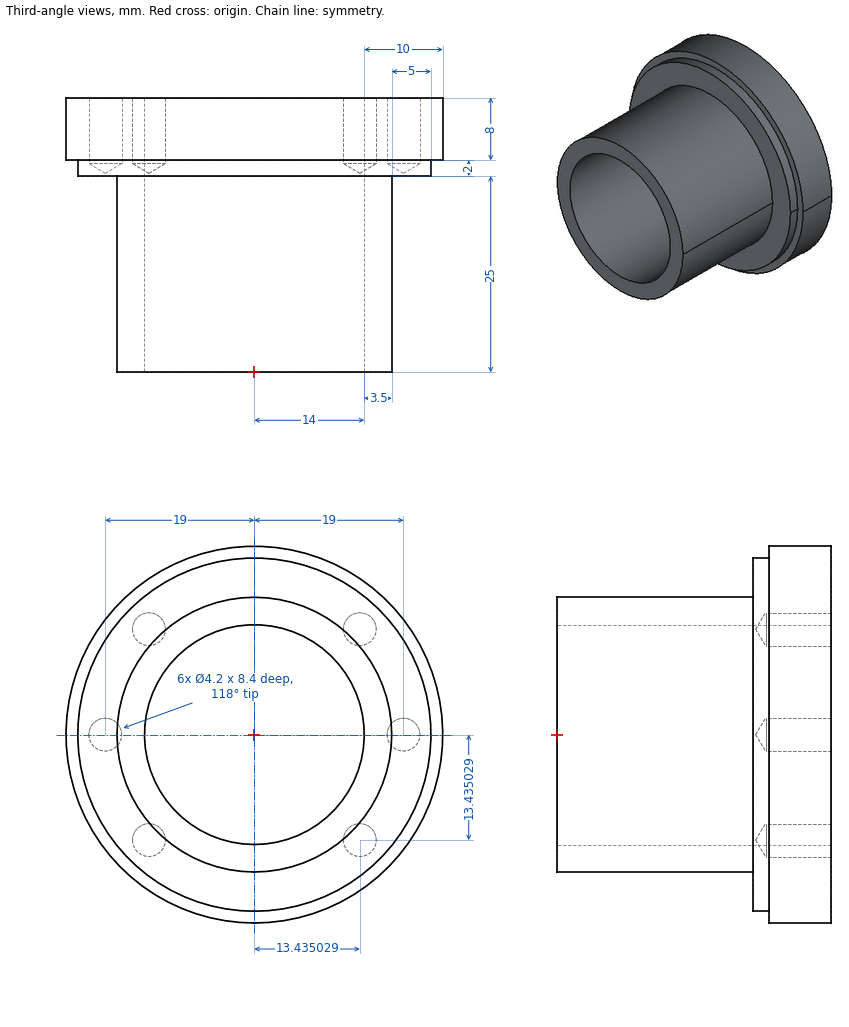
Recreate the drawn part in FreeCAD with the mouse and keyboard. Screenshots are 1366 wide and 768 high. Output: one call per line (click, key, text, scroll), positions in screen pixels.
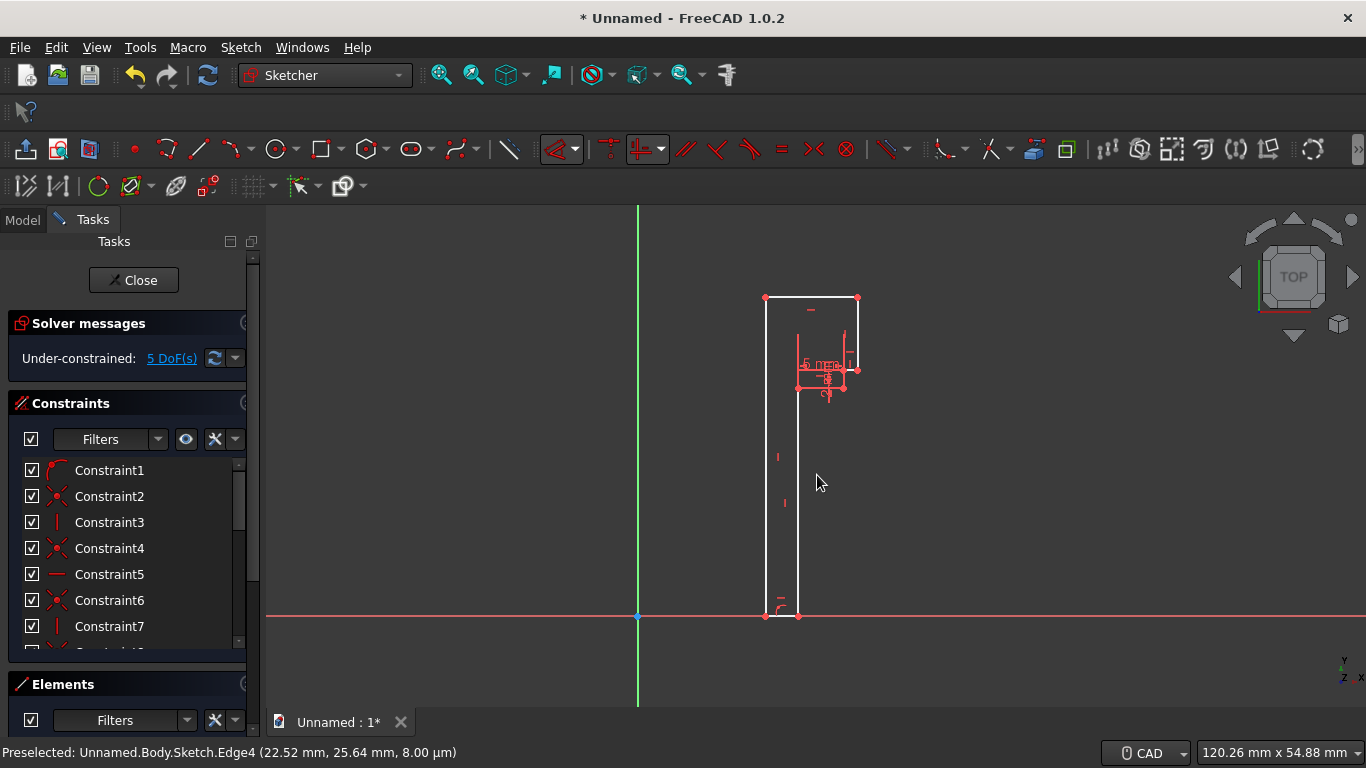
click(858, 348)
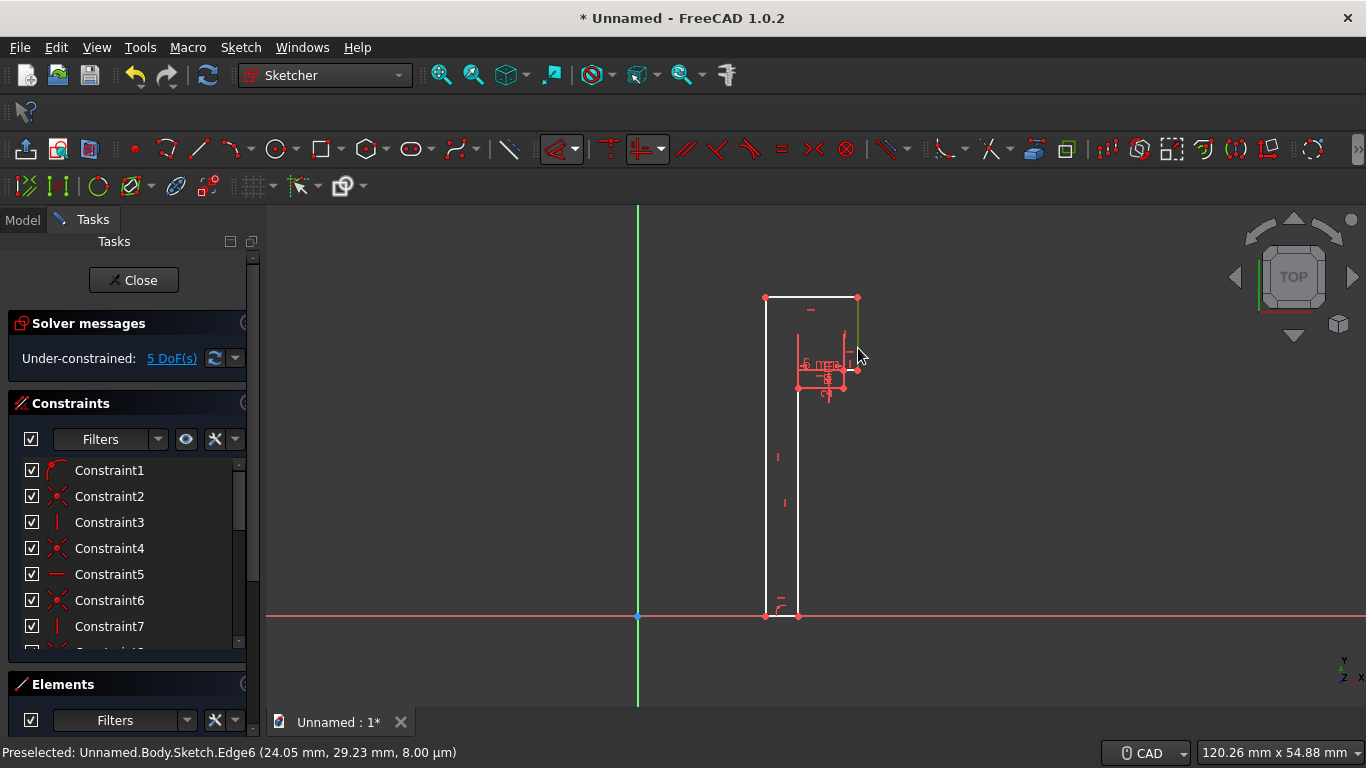
click(578, 150)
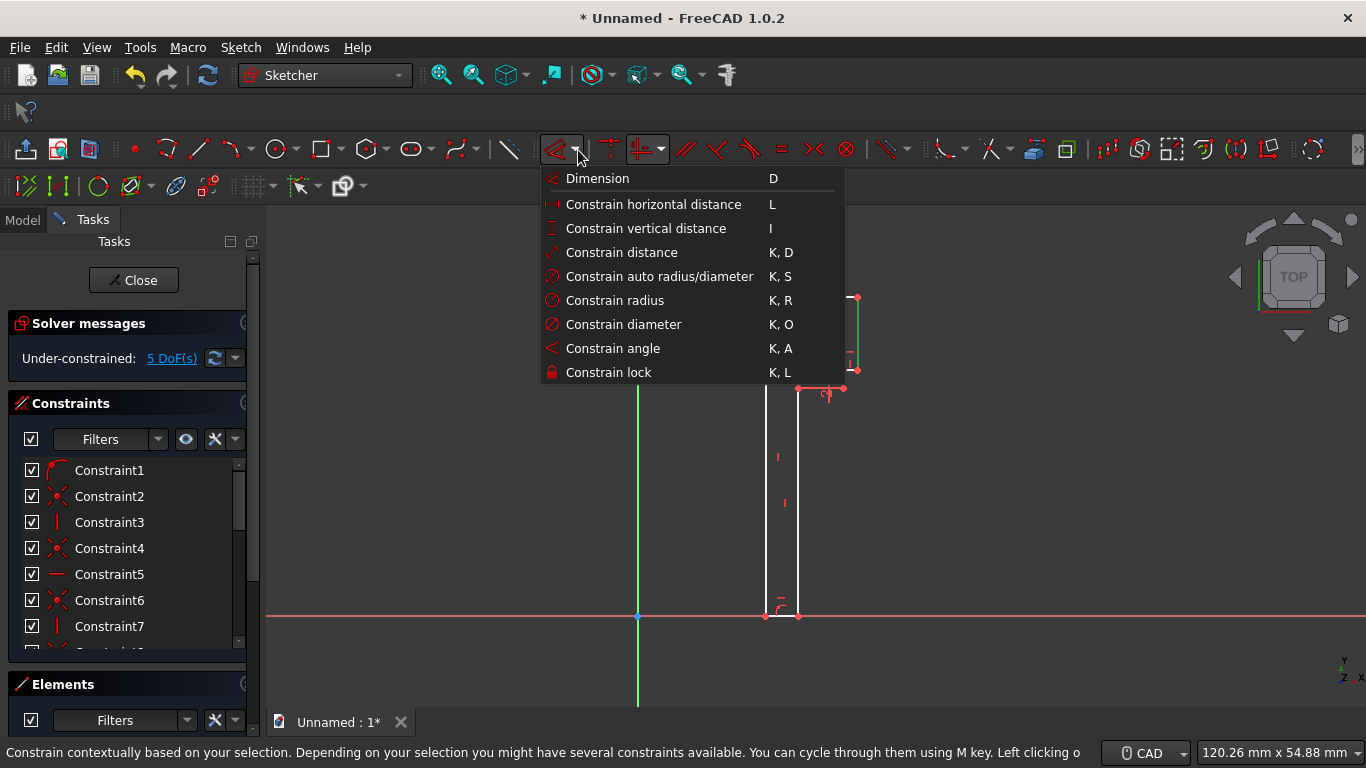
click(693, 228)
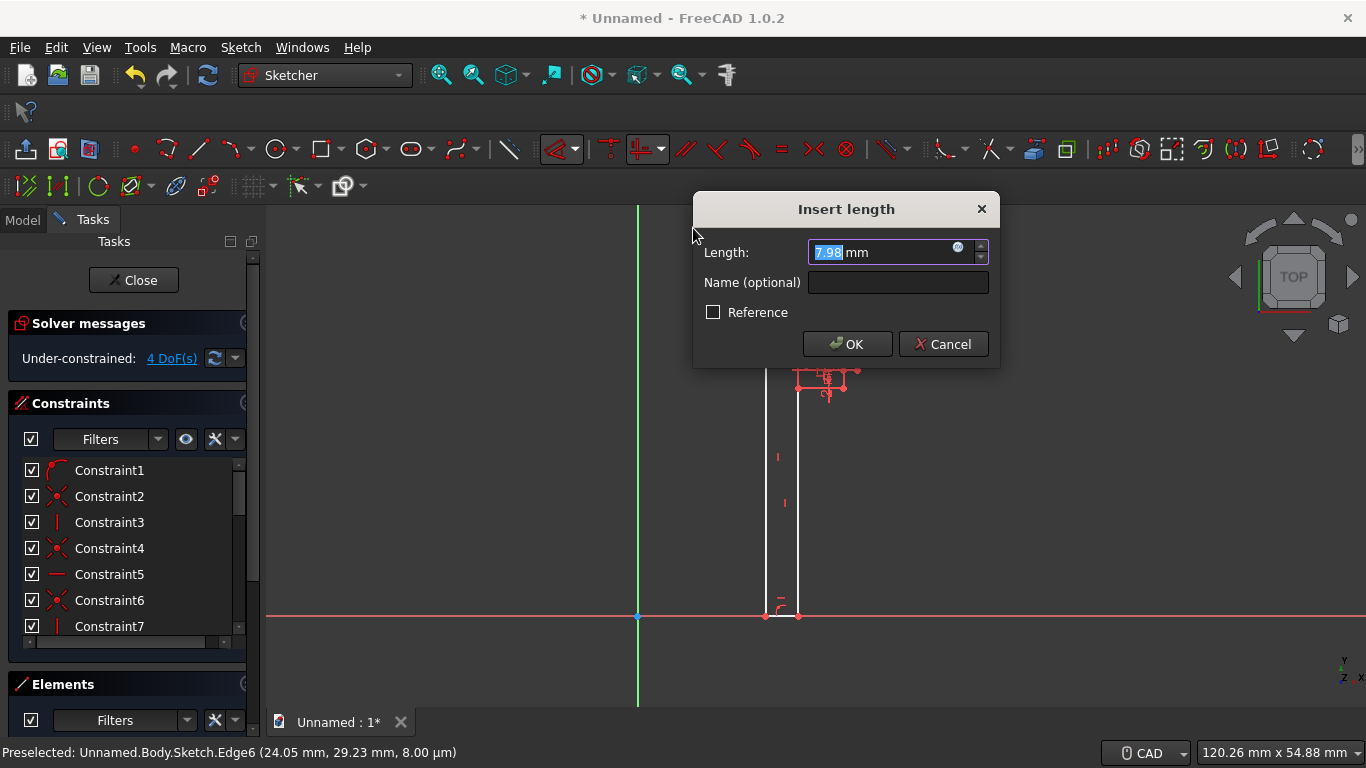
text(8)
key(Return)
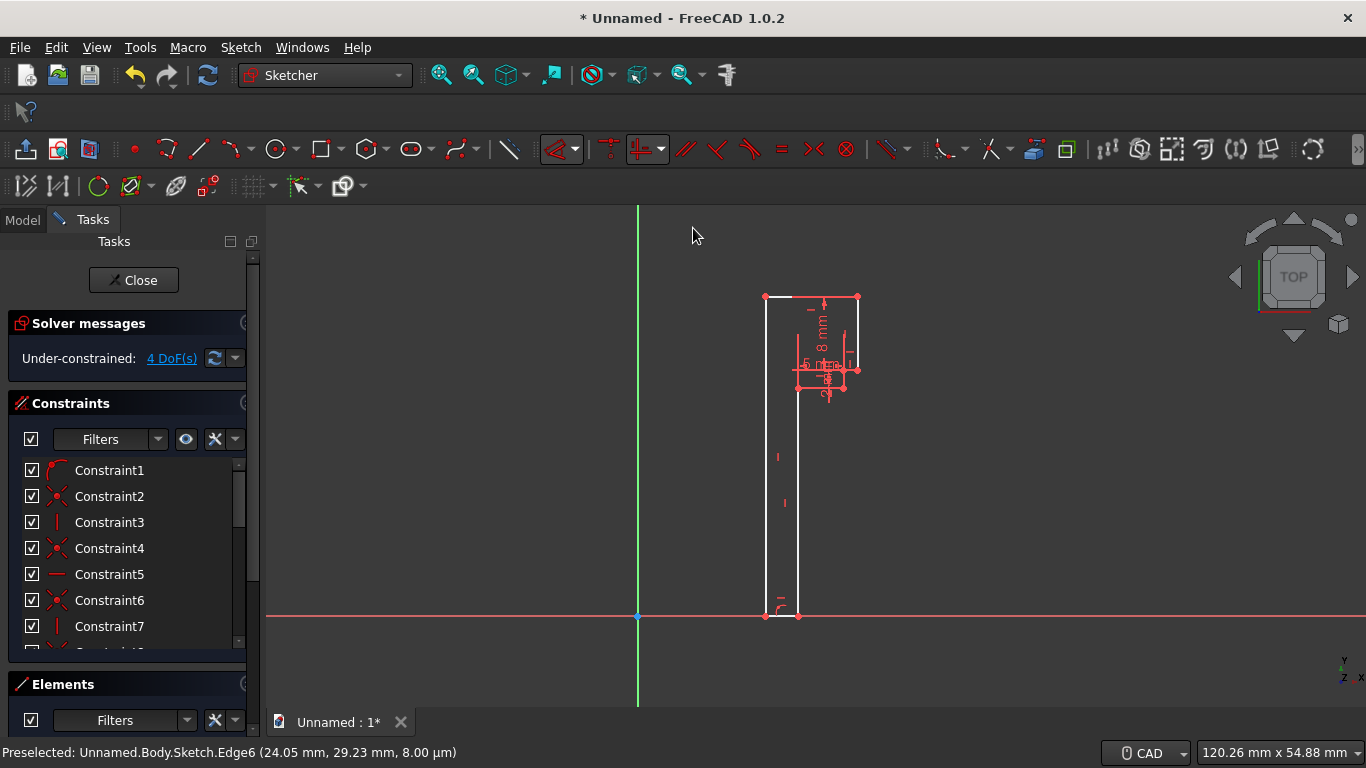
click(798, 548)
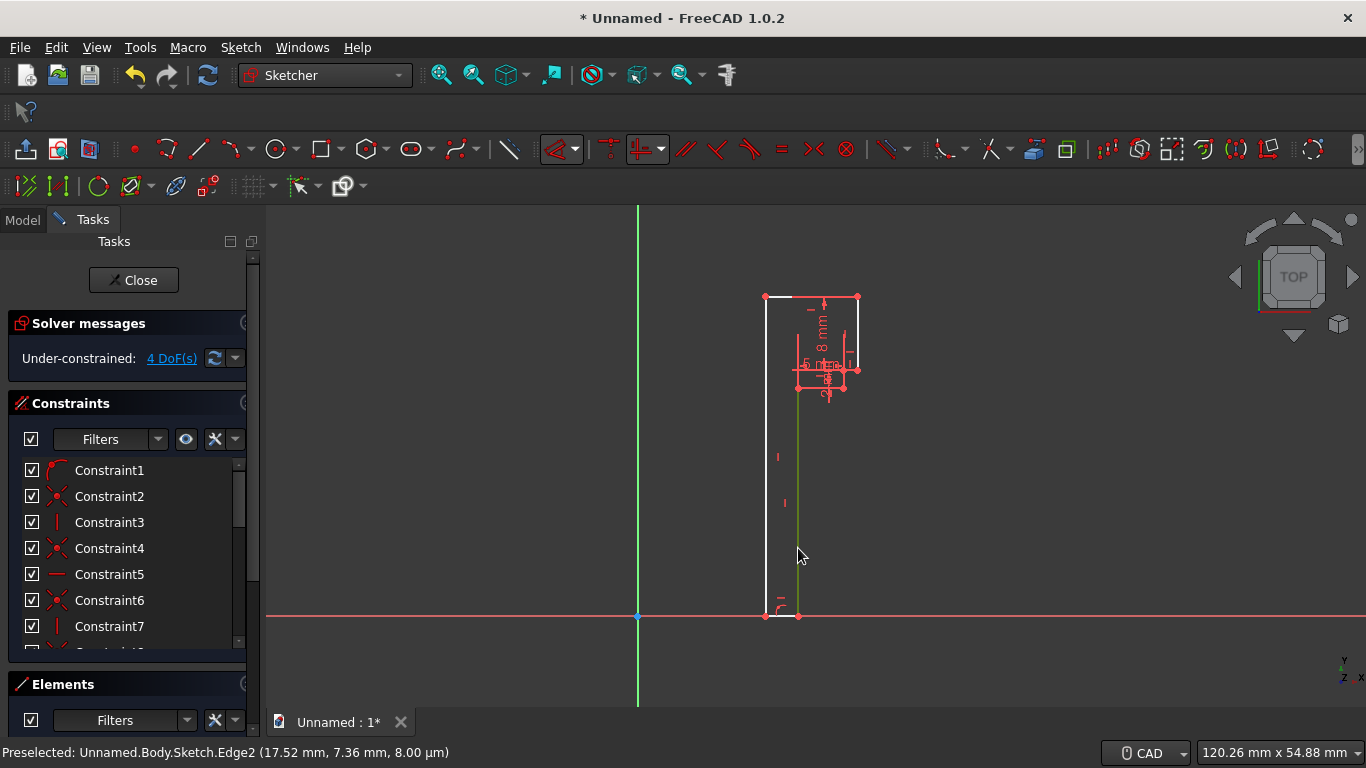
click(578, 150)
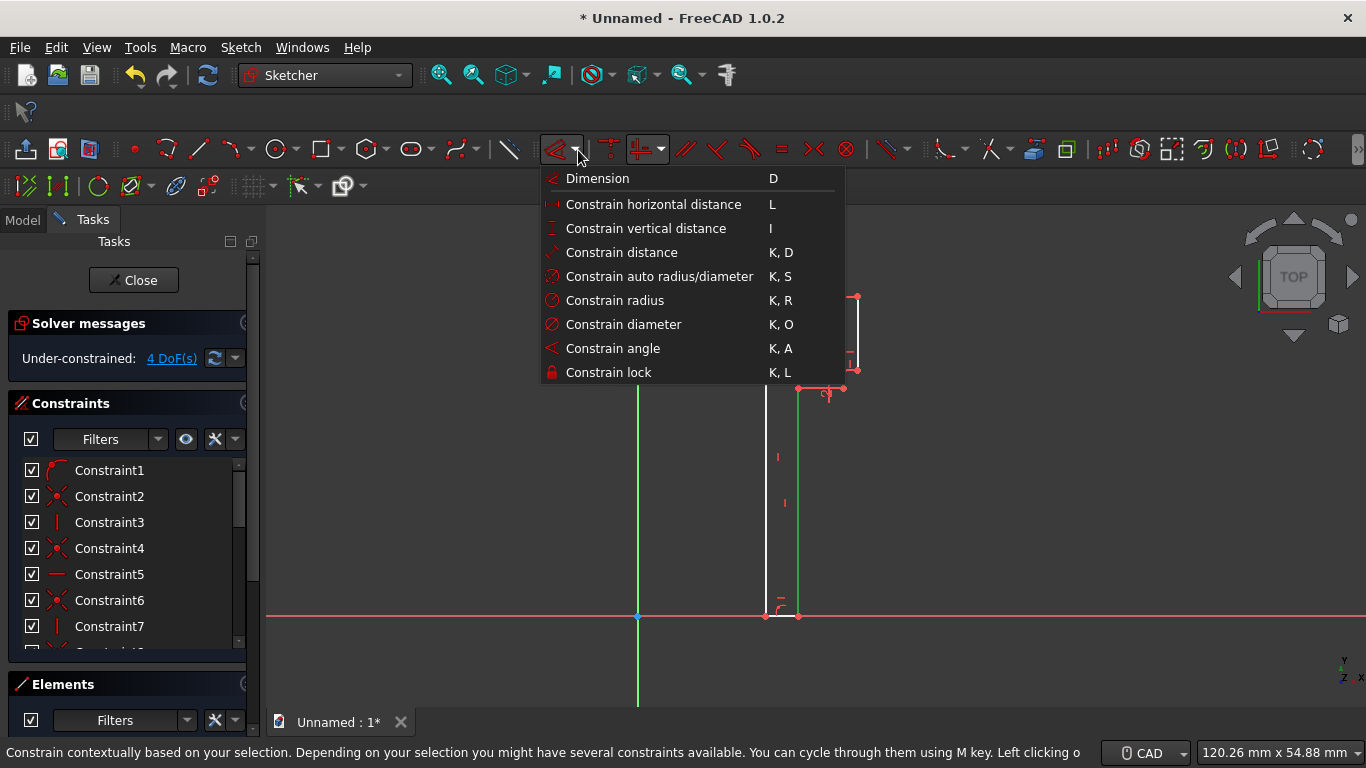
click(693, 228)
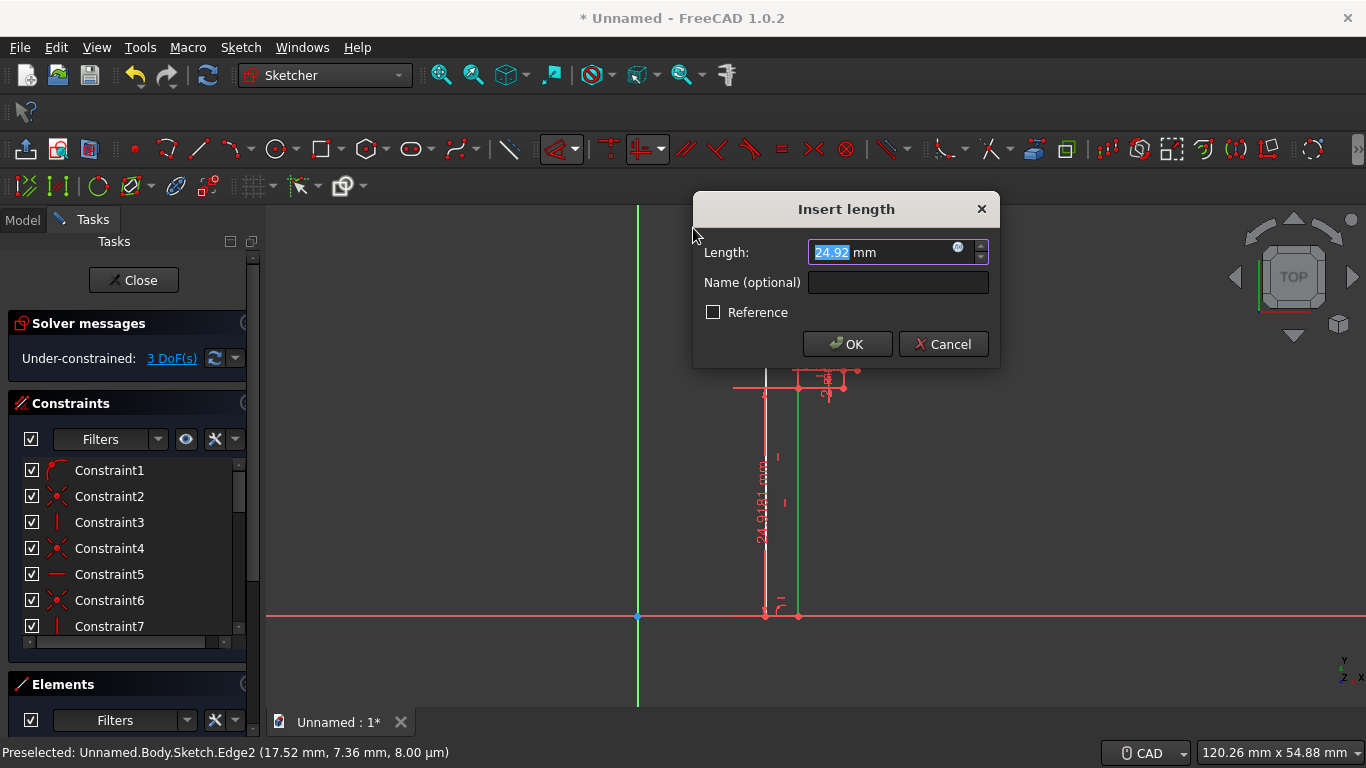
text(25)
key(Return)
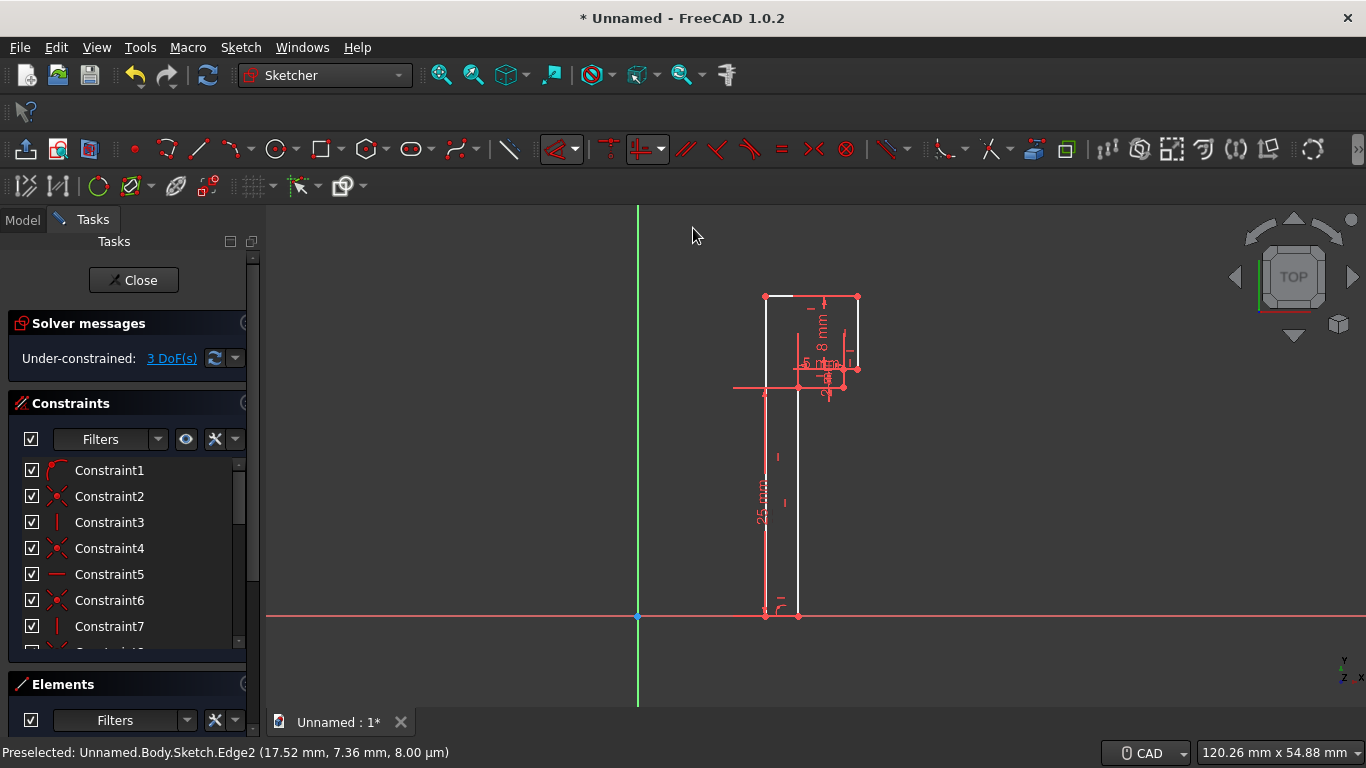
click(830, 296)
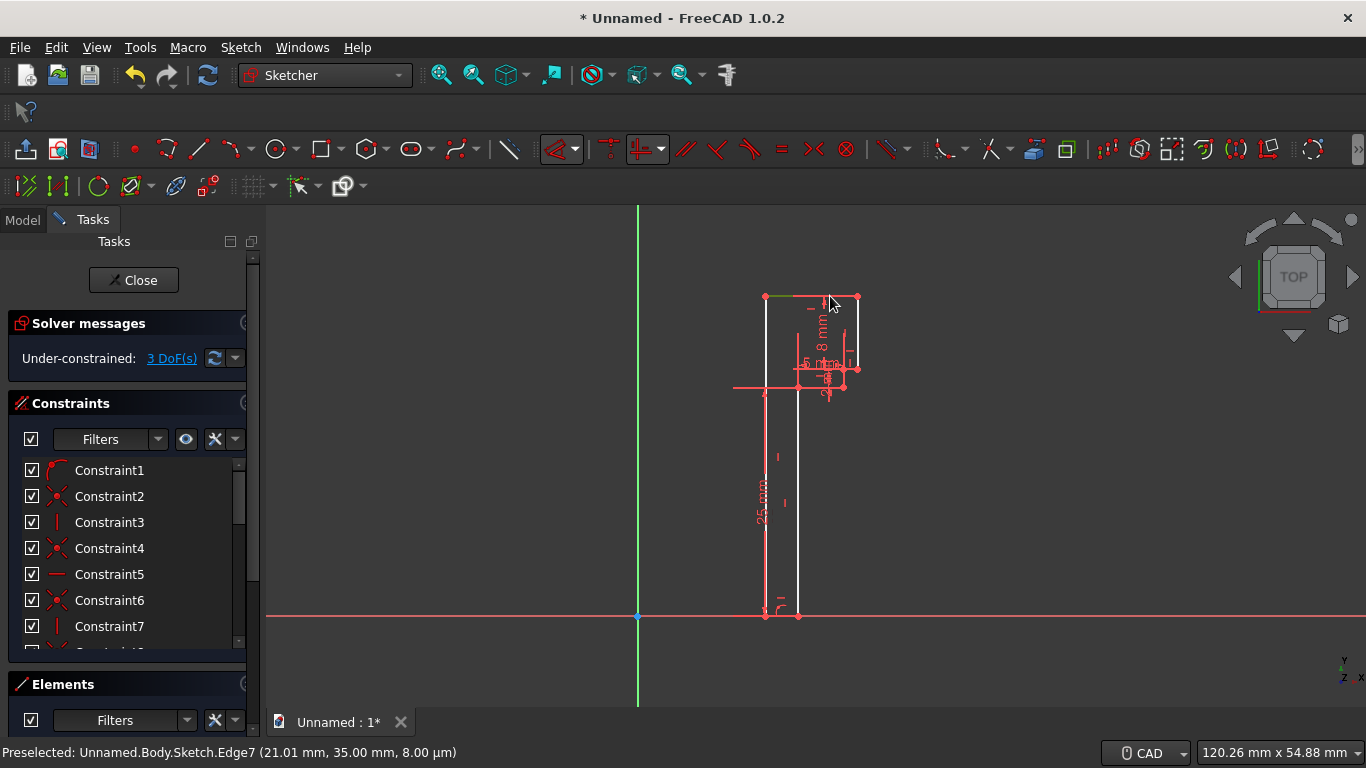
key(l)